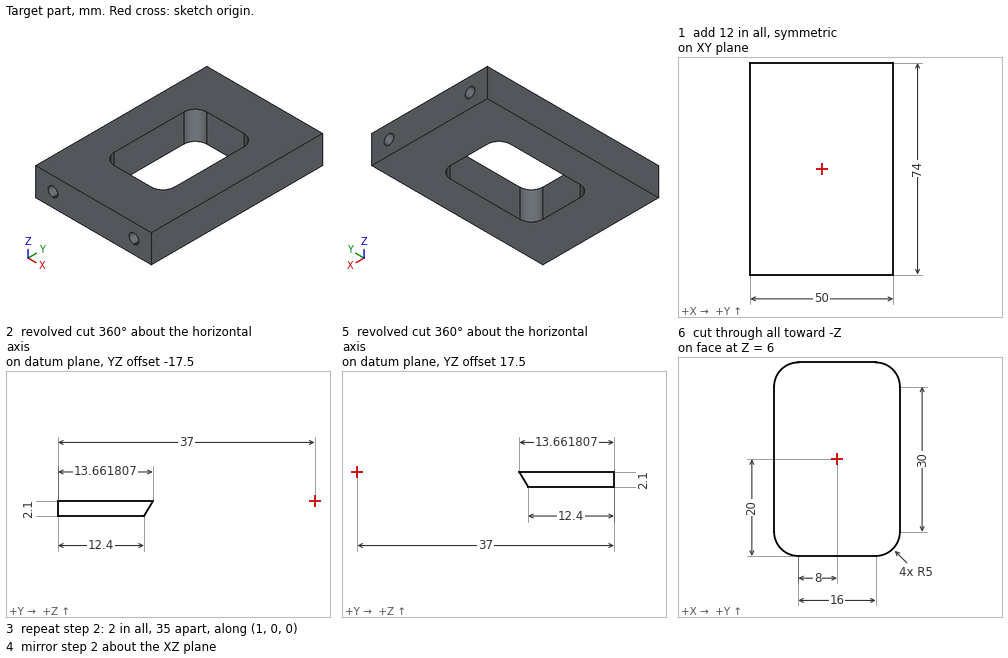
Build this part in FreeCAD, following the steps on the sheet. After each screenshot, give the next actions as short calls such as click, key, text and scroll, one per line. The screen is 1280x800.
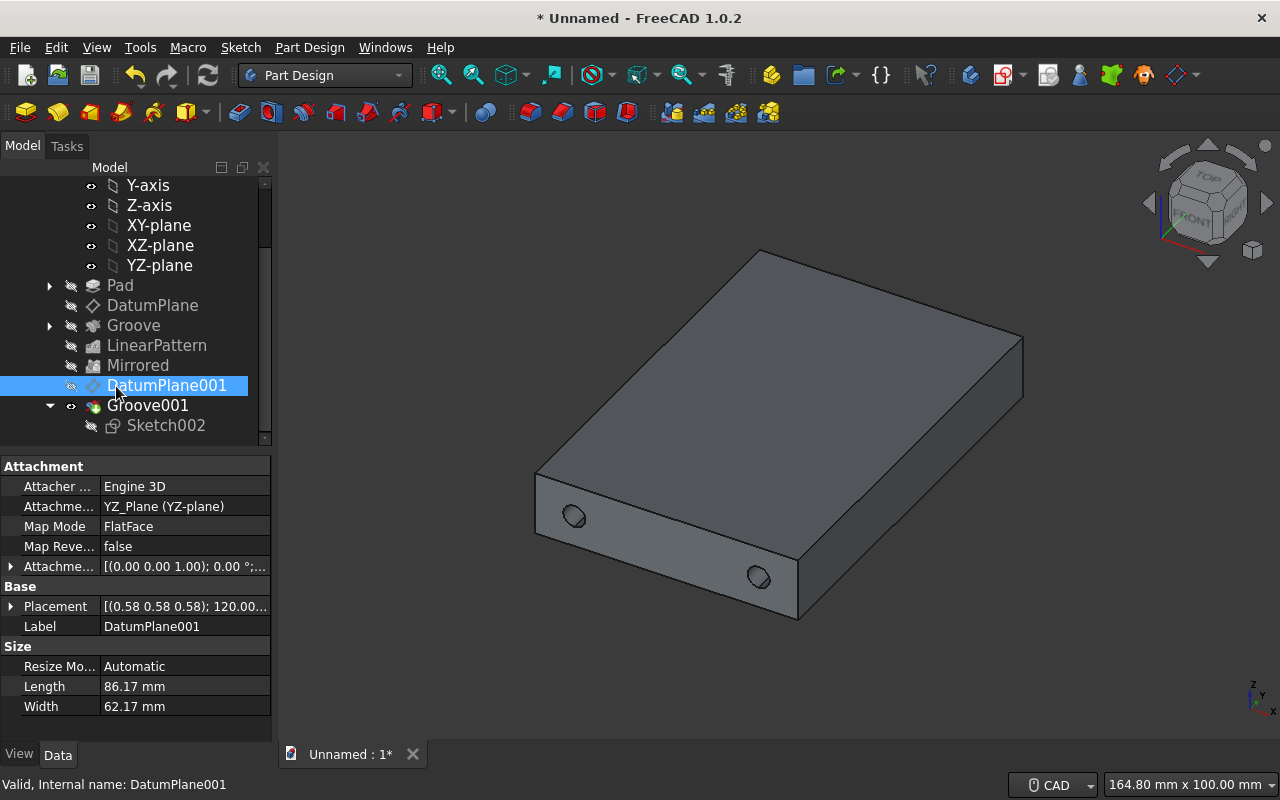
click(811, 372)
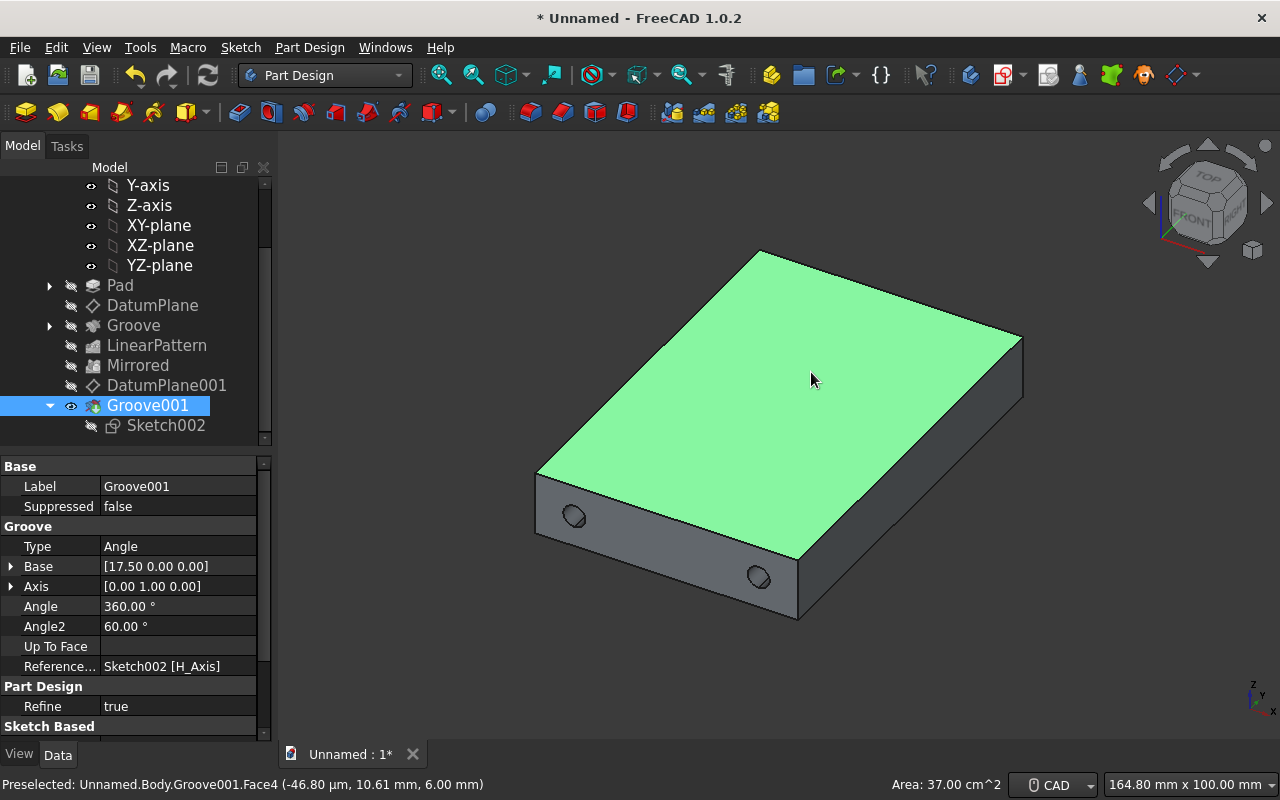
click(1004, 76)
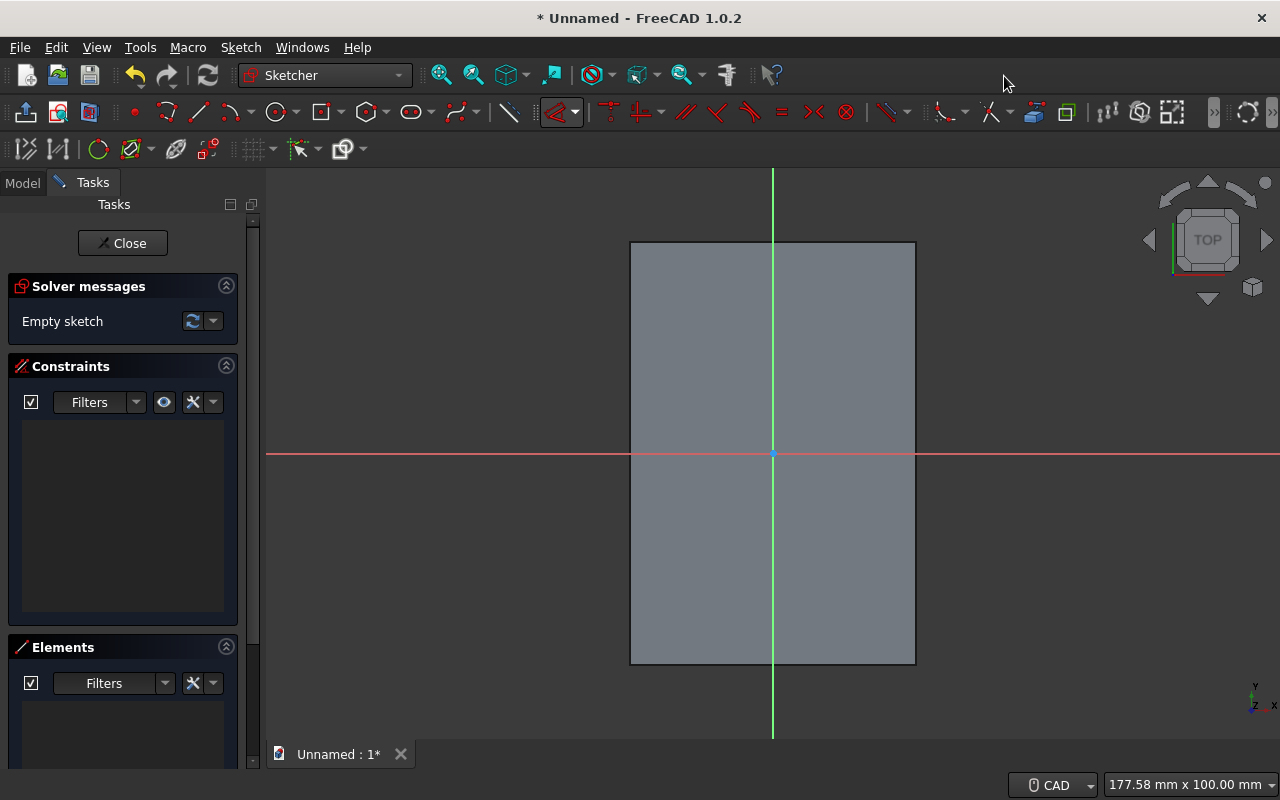
scroll(912, 454, up, 2)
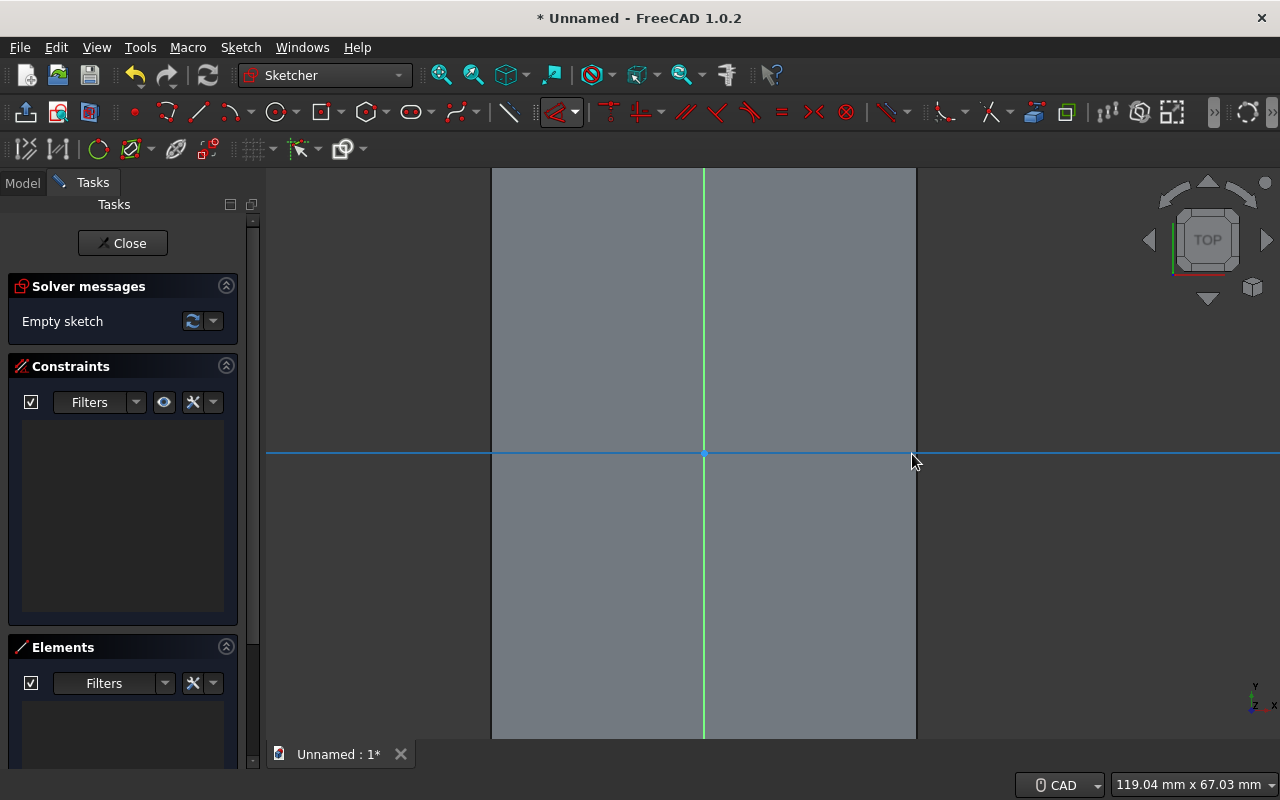
click(200, 112)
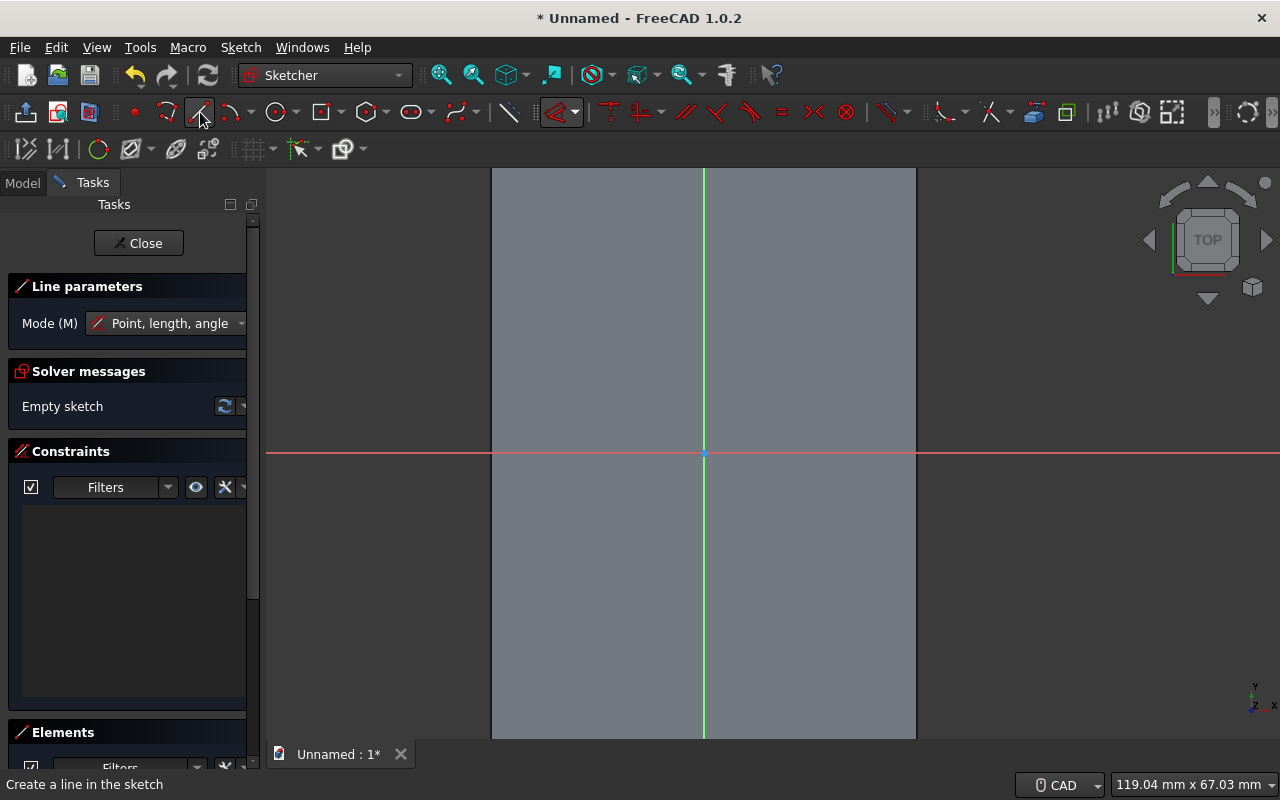
click(636, 623)
click(772, 623)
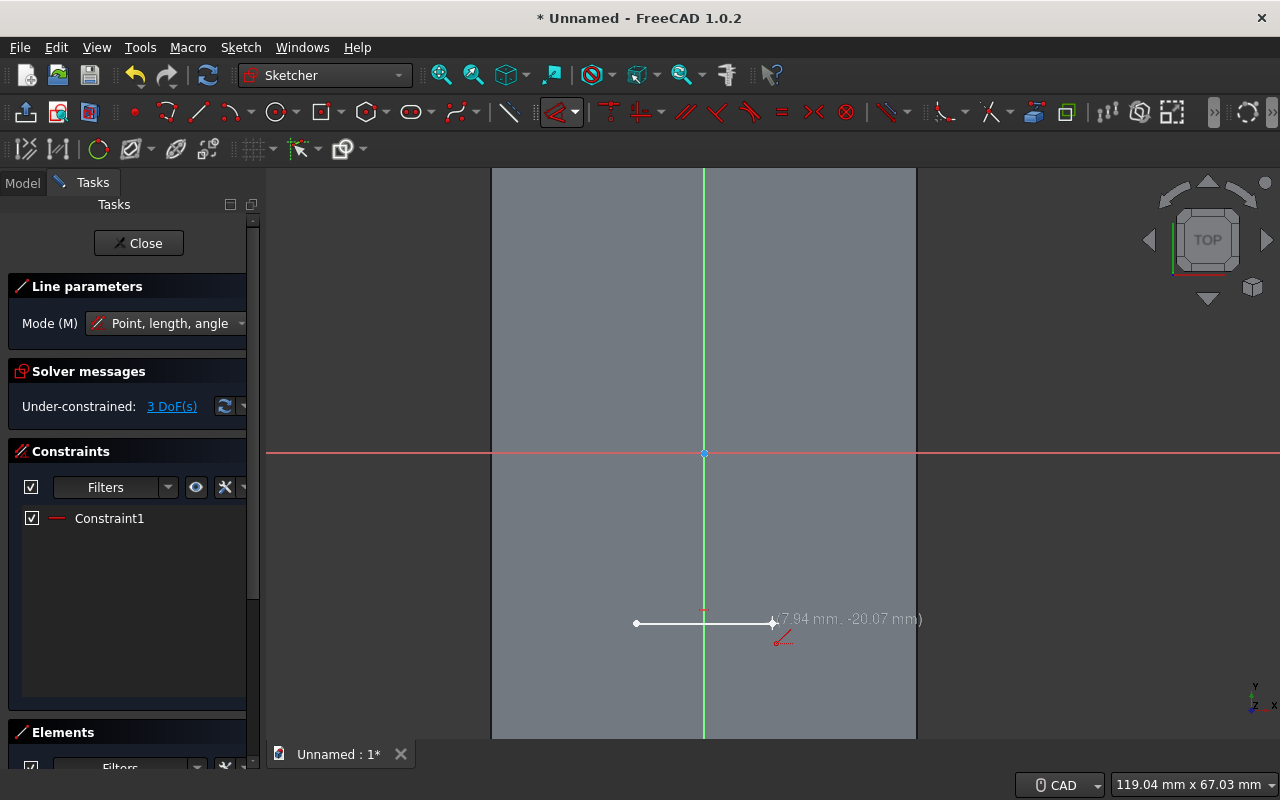
click(815, 581)
click(815, 325)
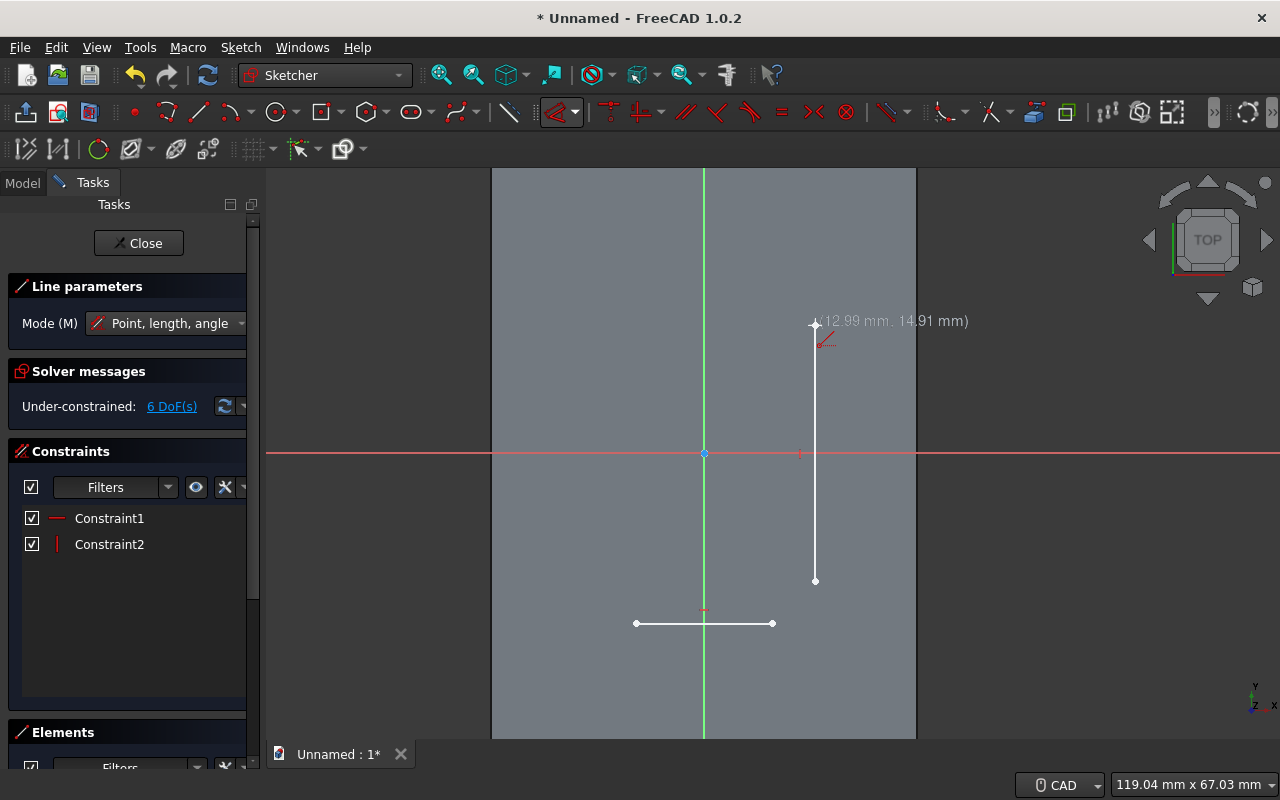
click(772, 283)
click(636, 283)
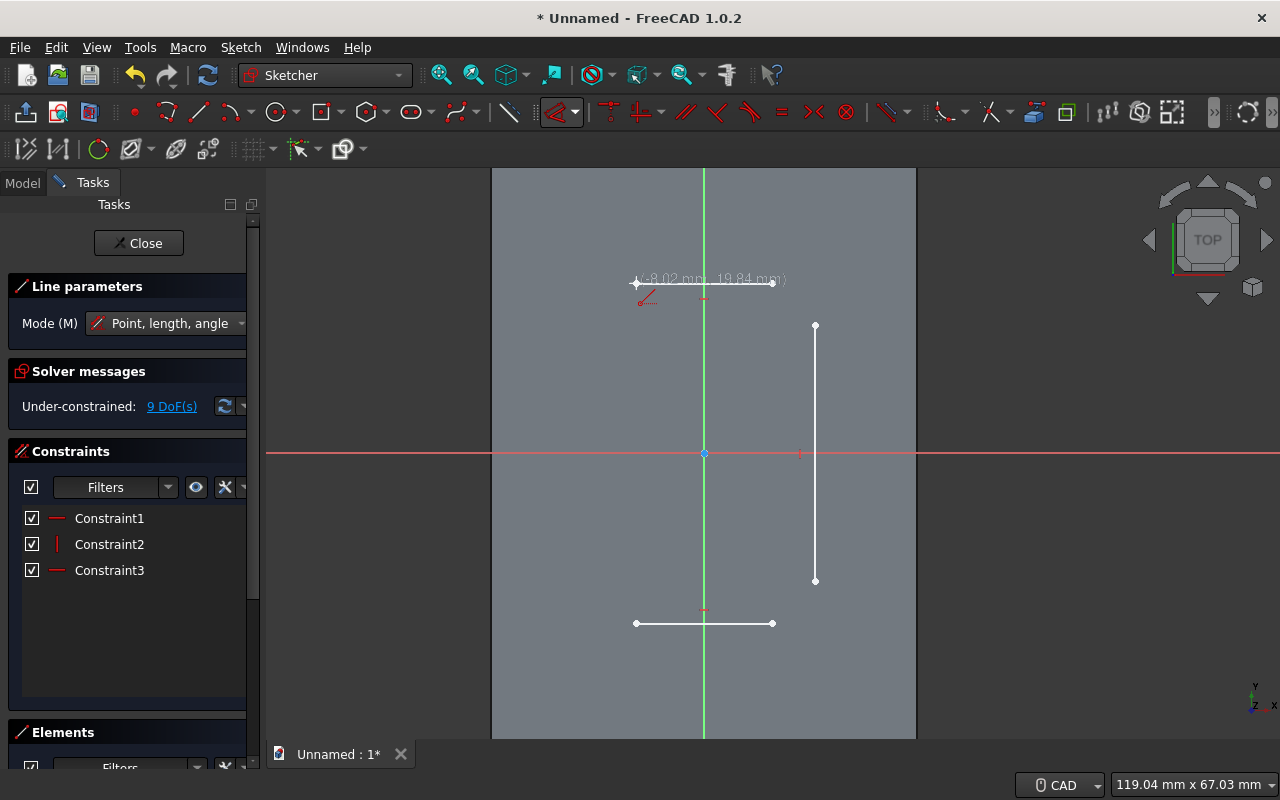
click(594, 325)
click(594, 581)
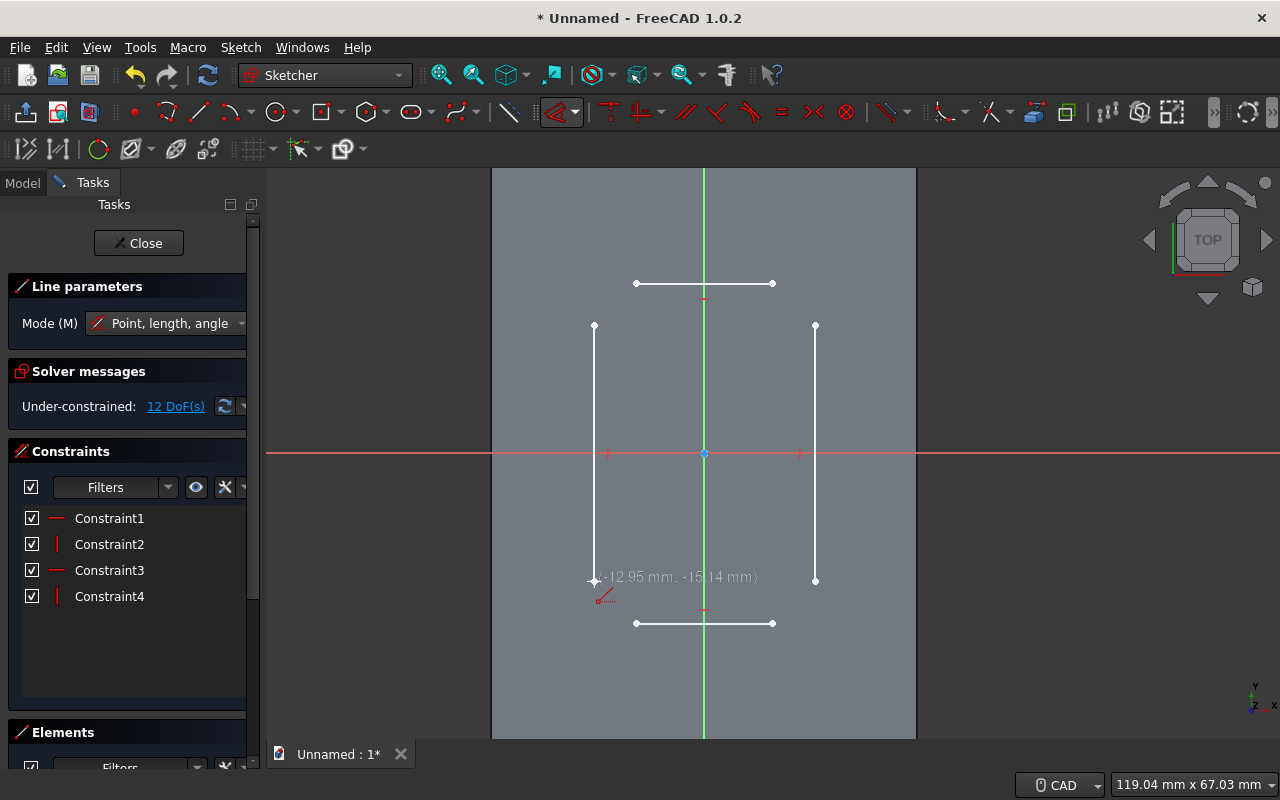
key(g)
key(3)
key(a)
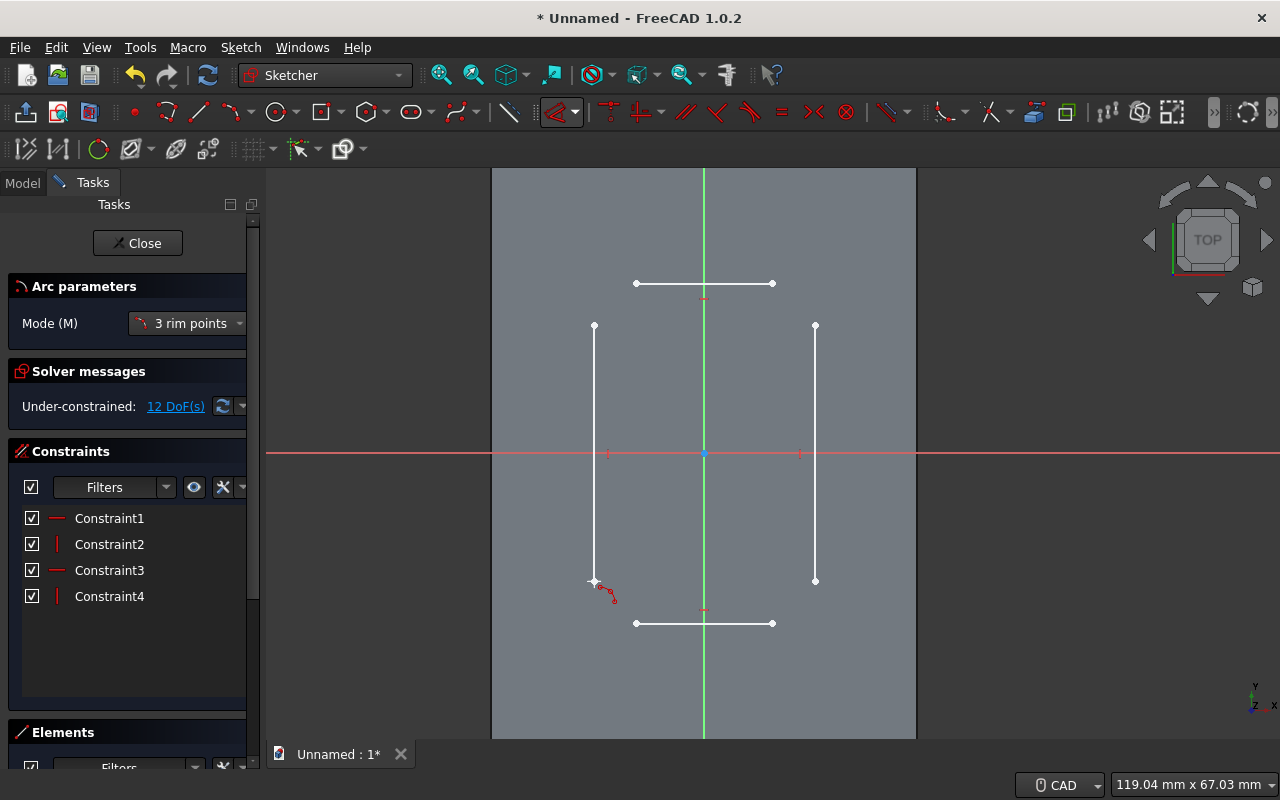
click(772, 624)
click(815, 582)